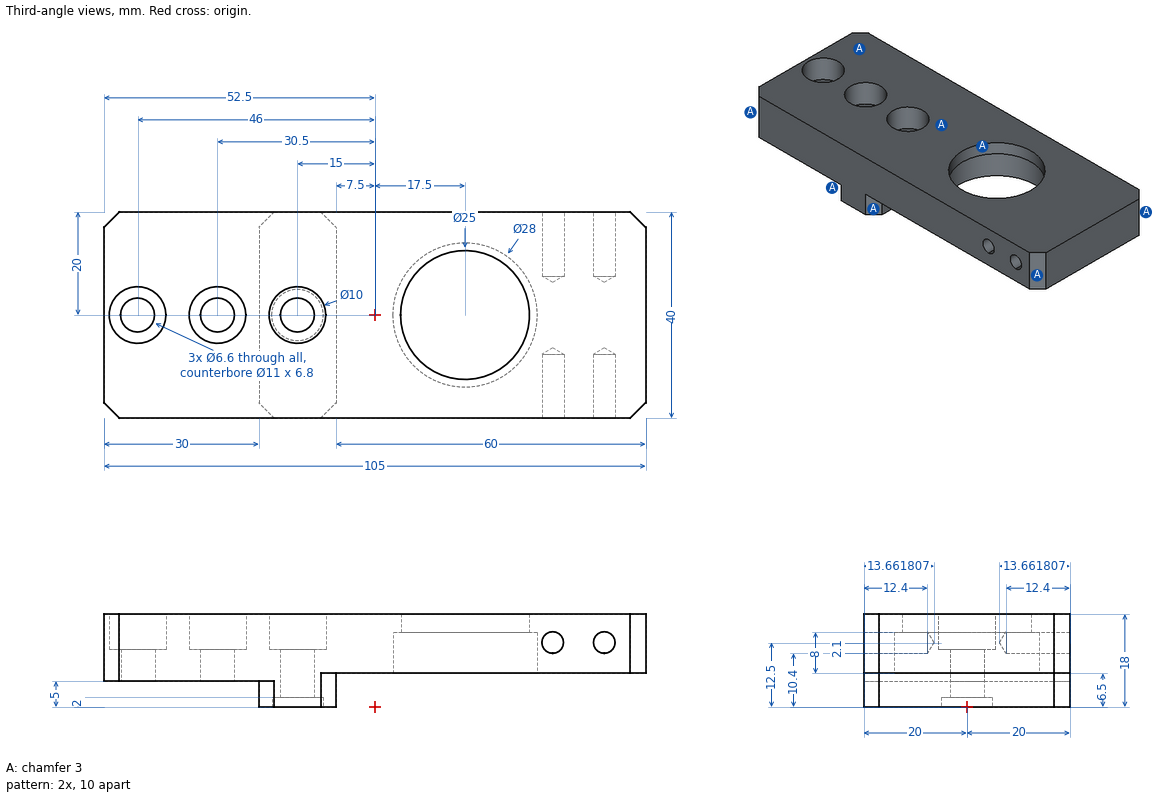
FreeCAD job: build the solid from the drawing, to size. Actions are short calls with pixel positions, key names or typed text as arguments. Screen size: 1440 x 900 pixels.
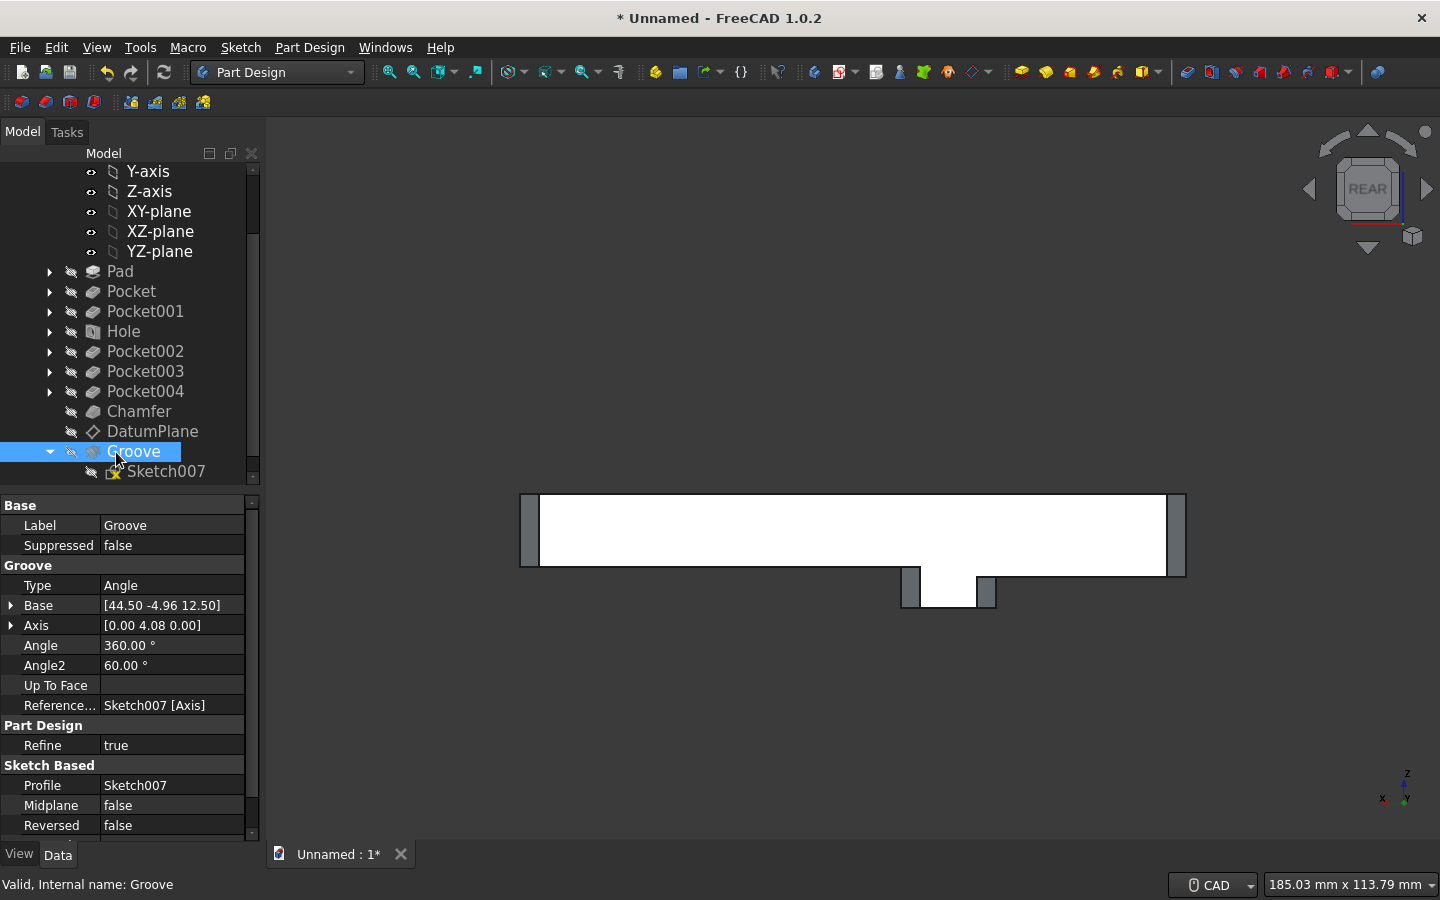
click(132, 102)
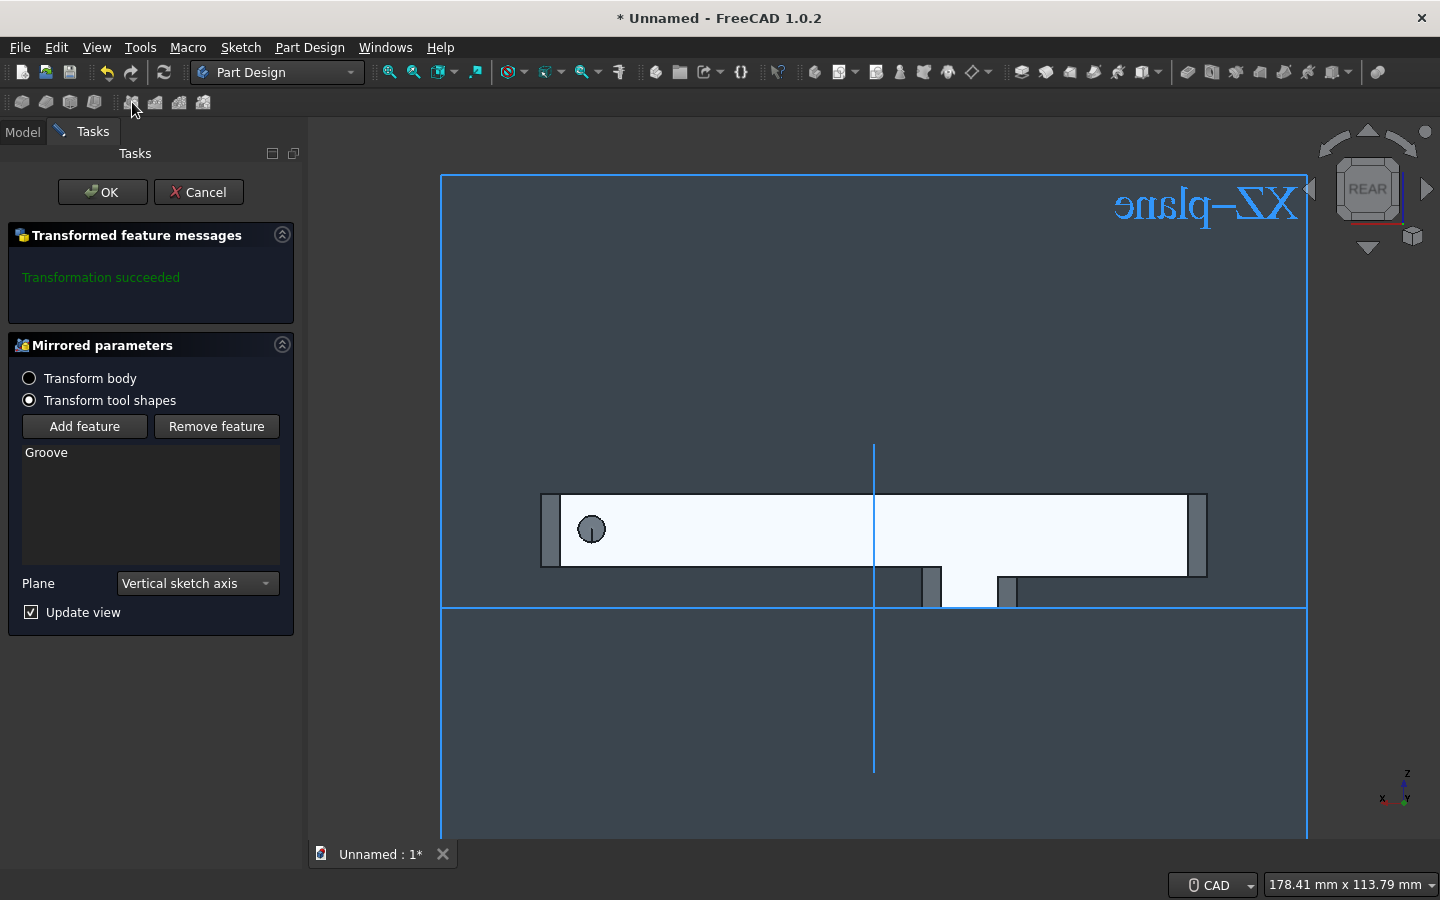
click(198, 584)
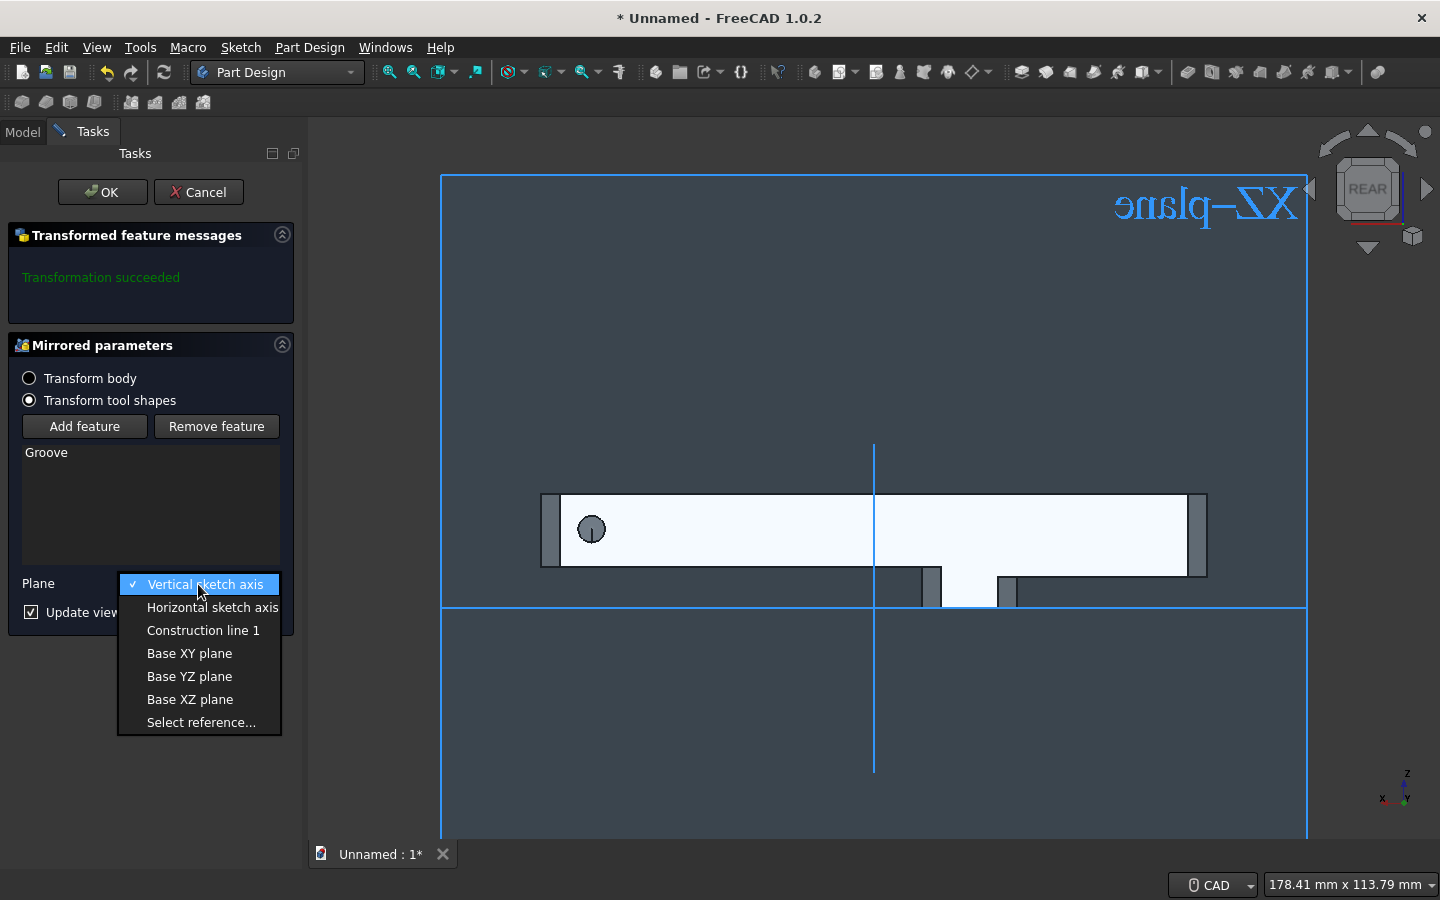
click(198, 700)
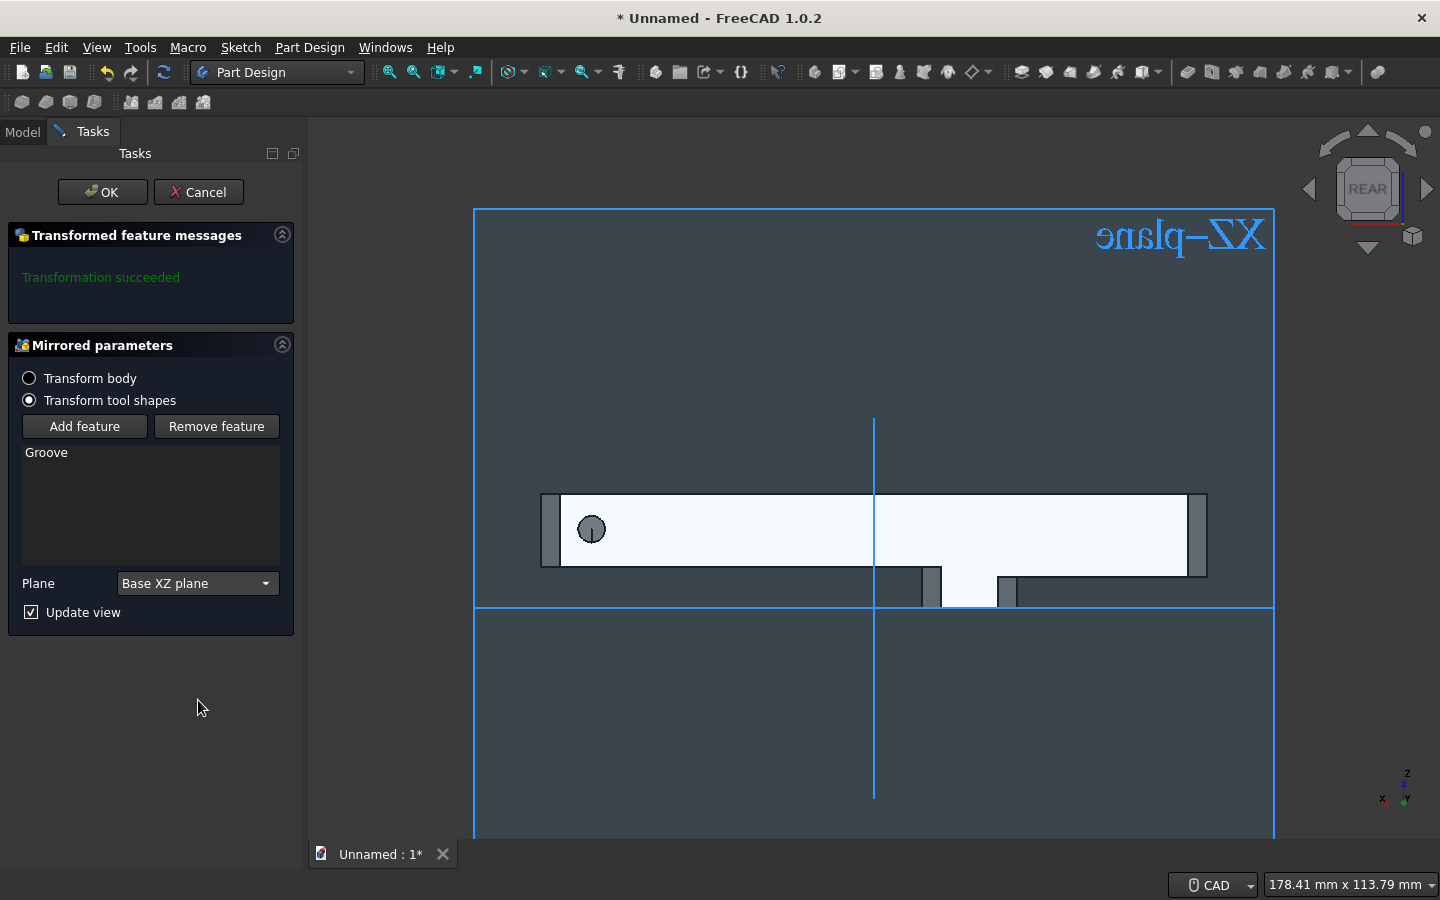
click(103, 192)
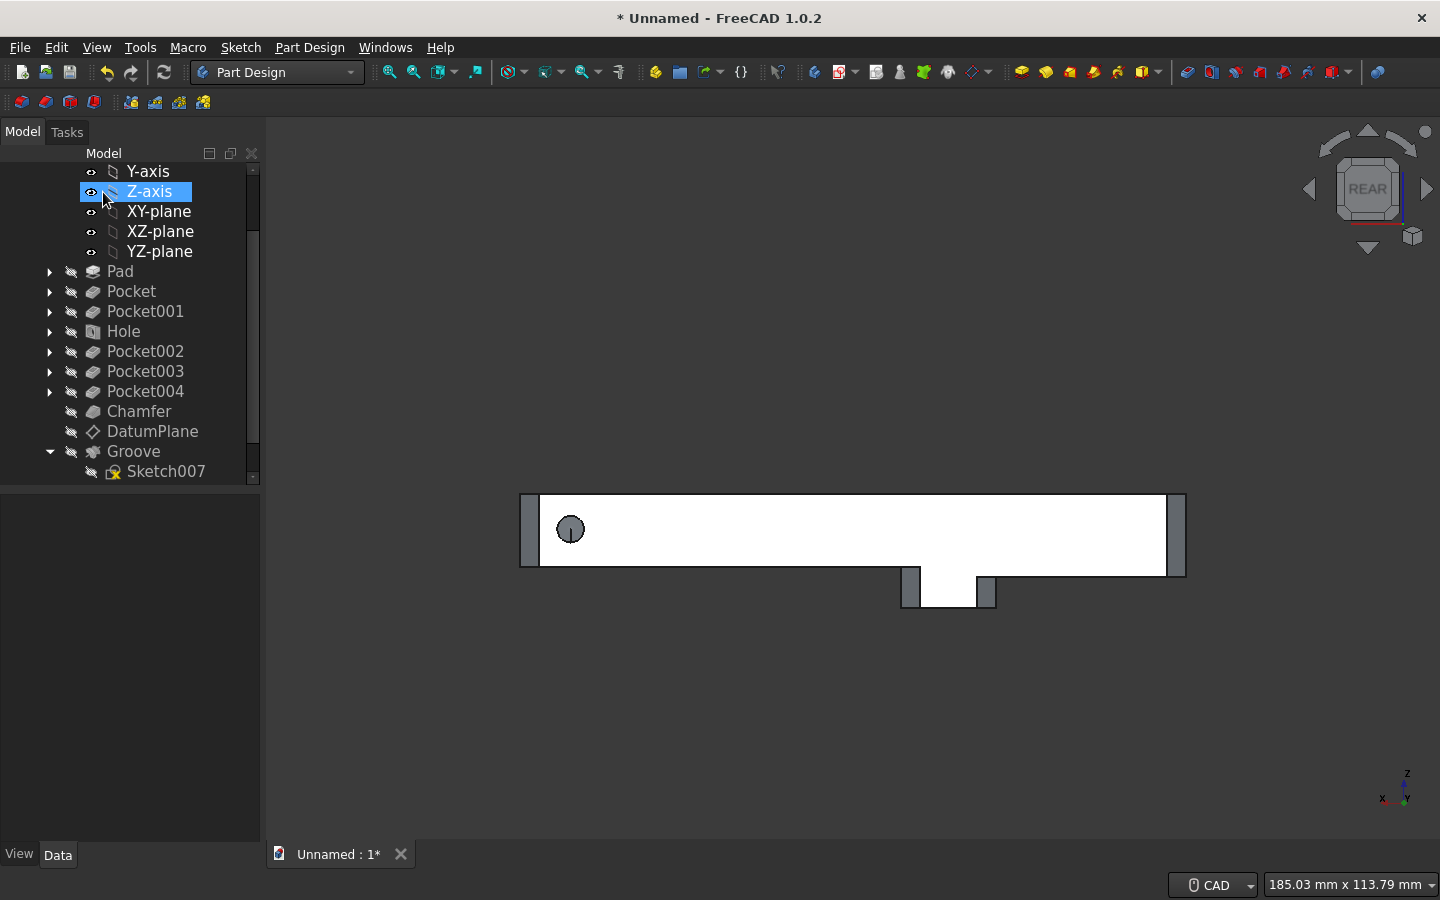
scroll(160, 327, down, 3)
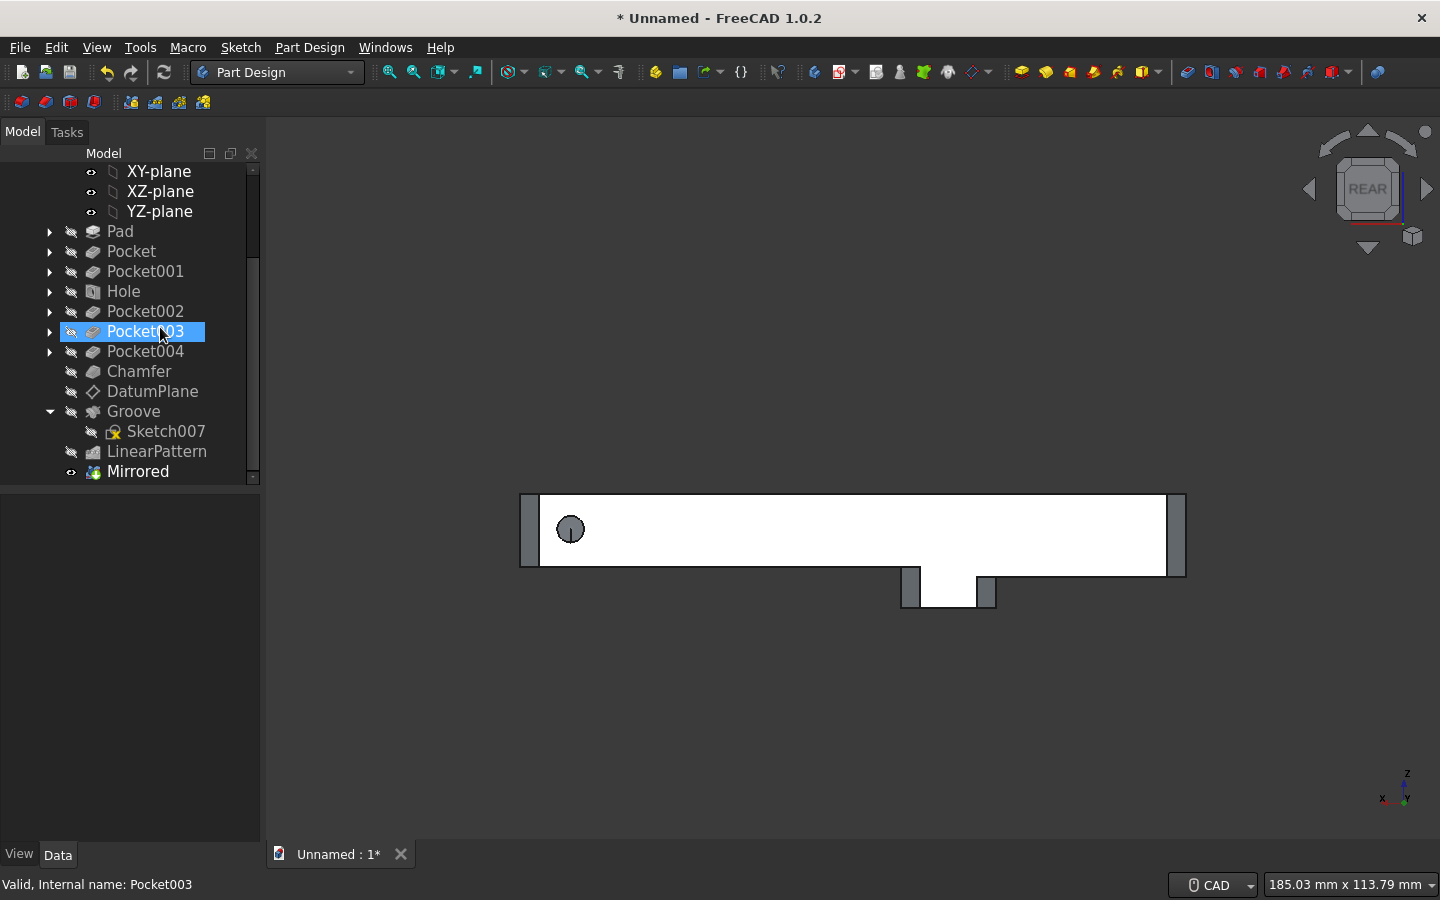
scroll(160, 327, up, 15)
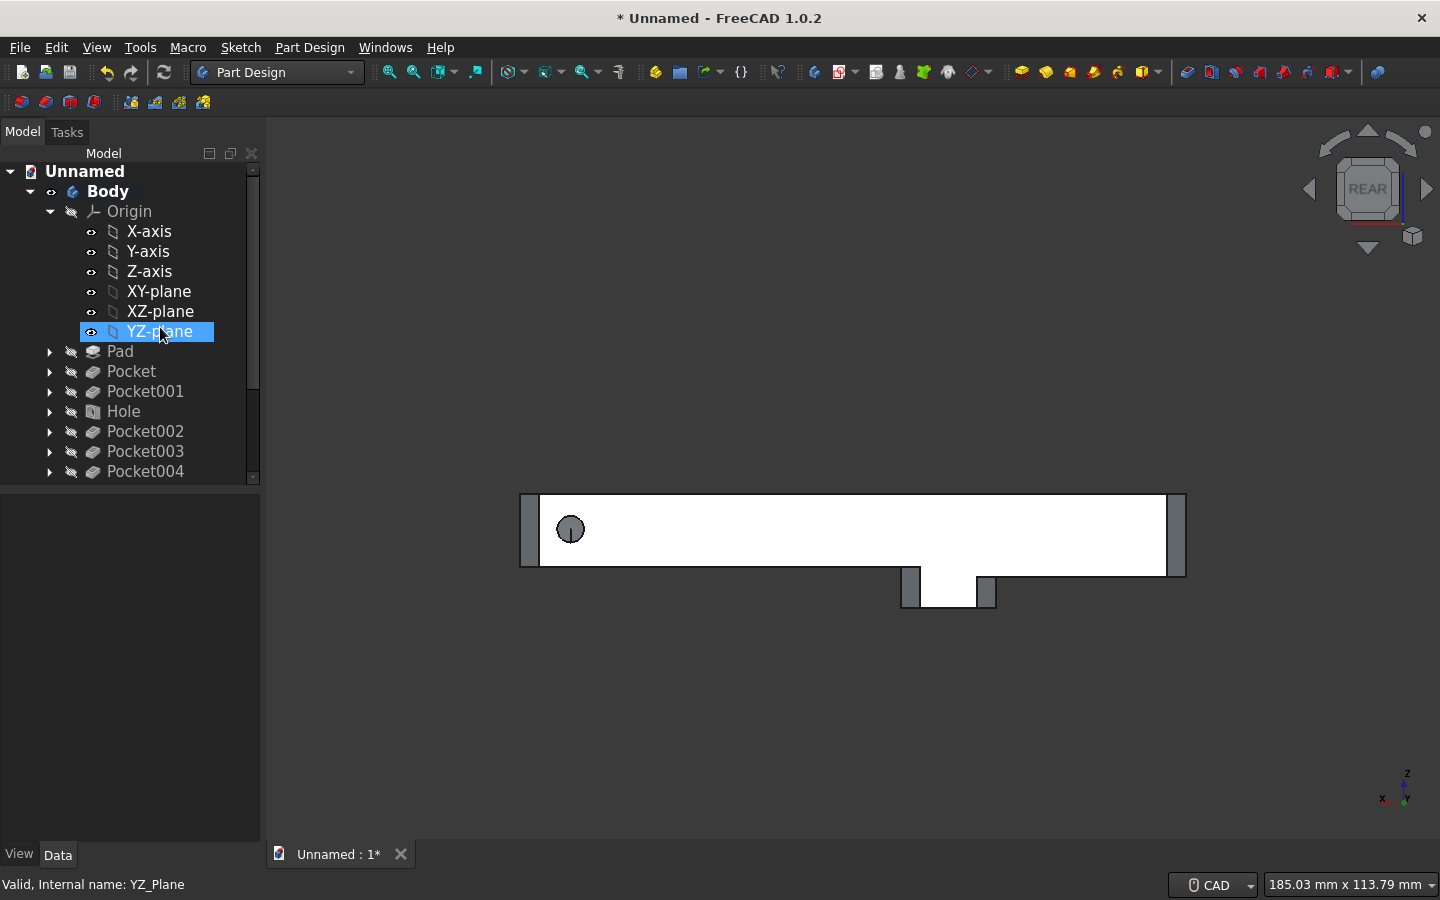
click(136, 332)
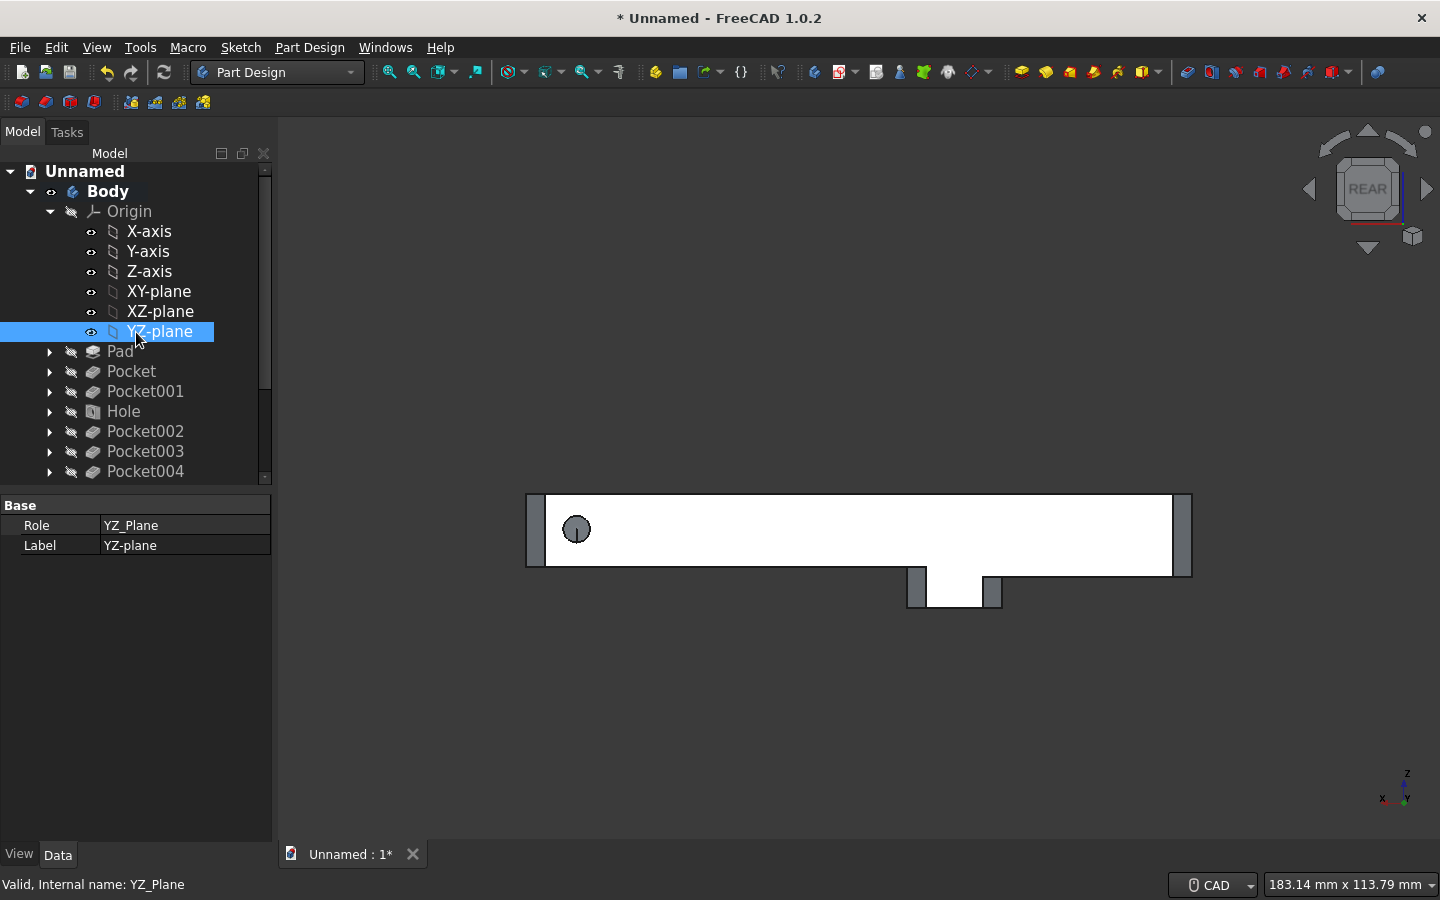
click(972, 72)